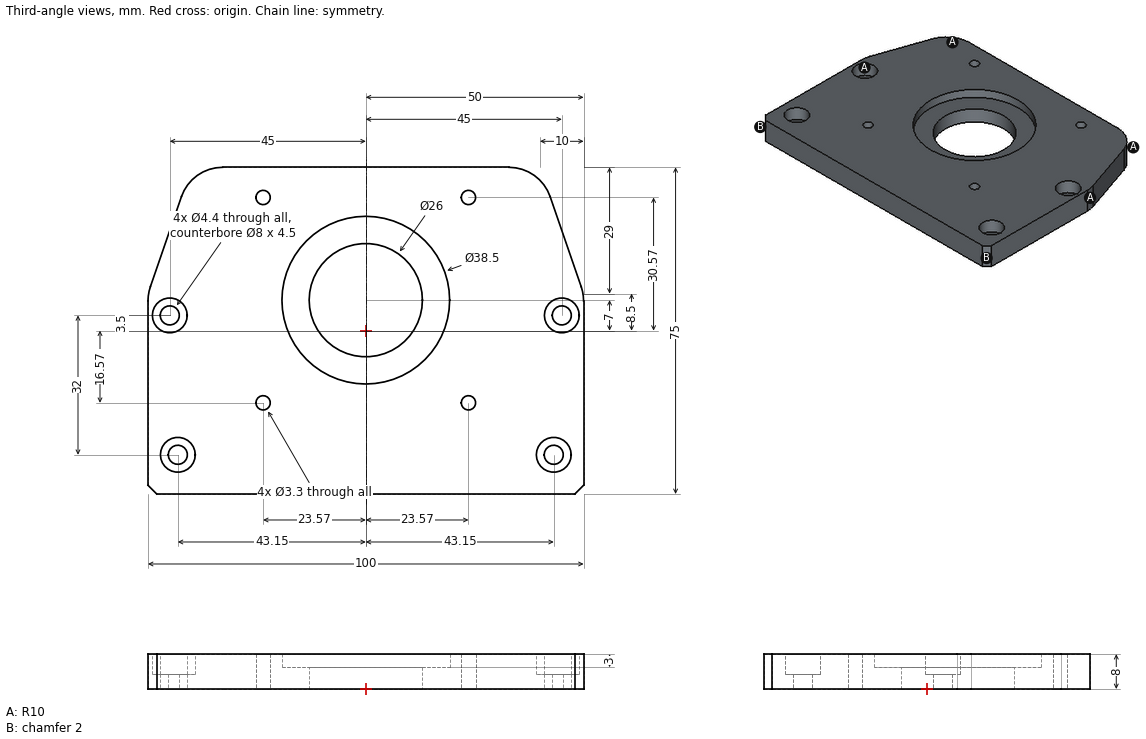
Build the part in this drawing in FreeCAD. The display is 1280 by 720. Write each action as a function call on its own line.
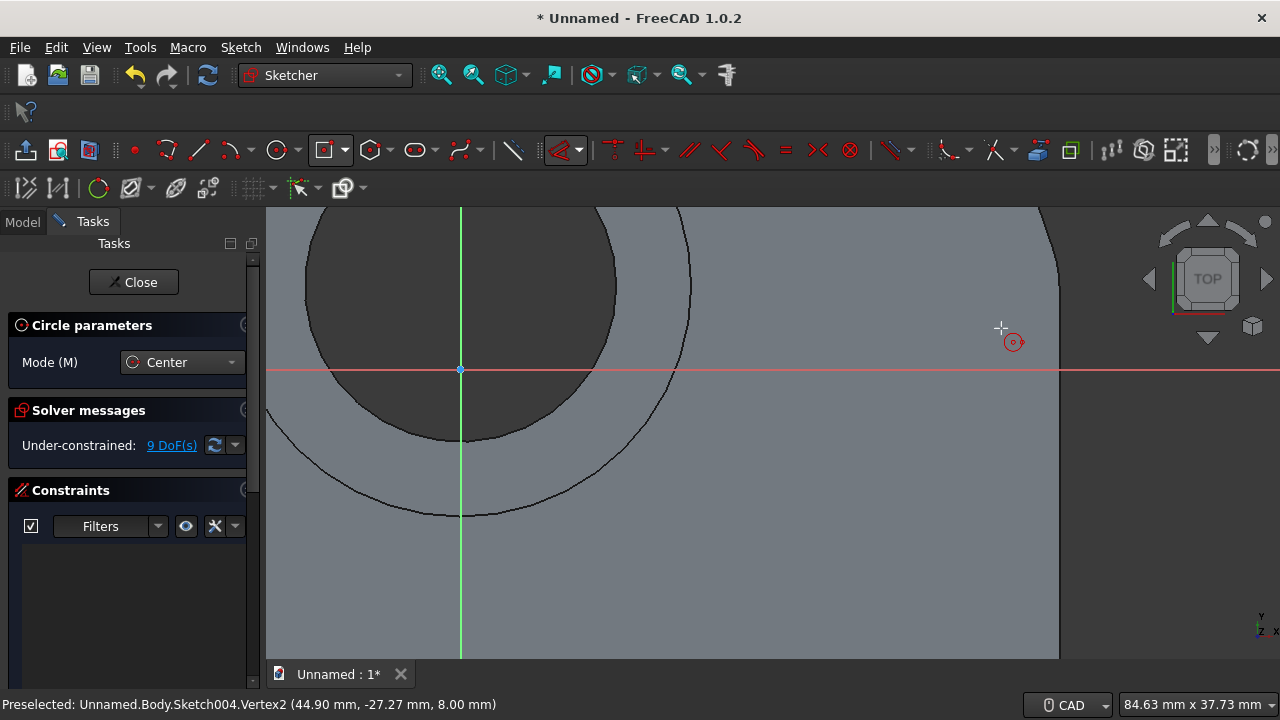
click(1000, 328)
click(1018, 309)
key(Escape)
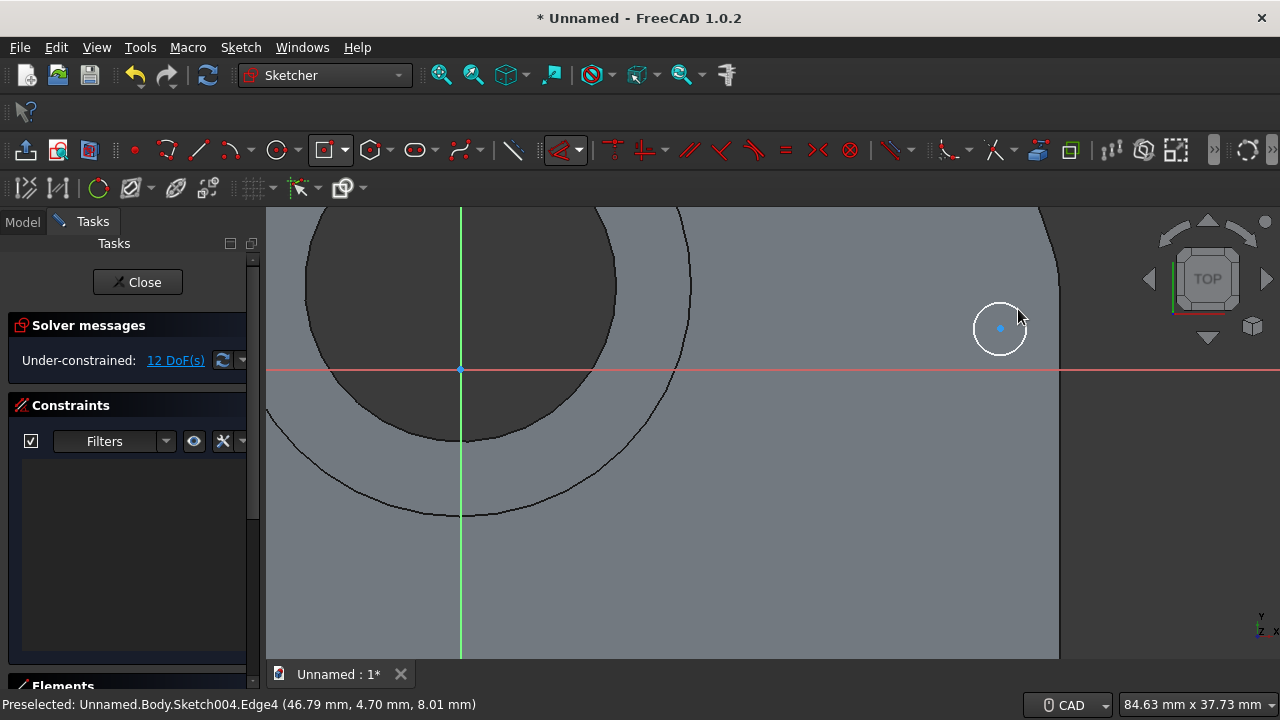
scroll(1001, 328, down, 3)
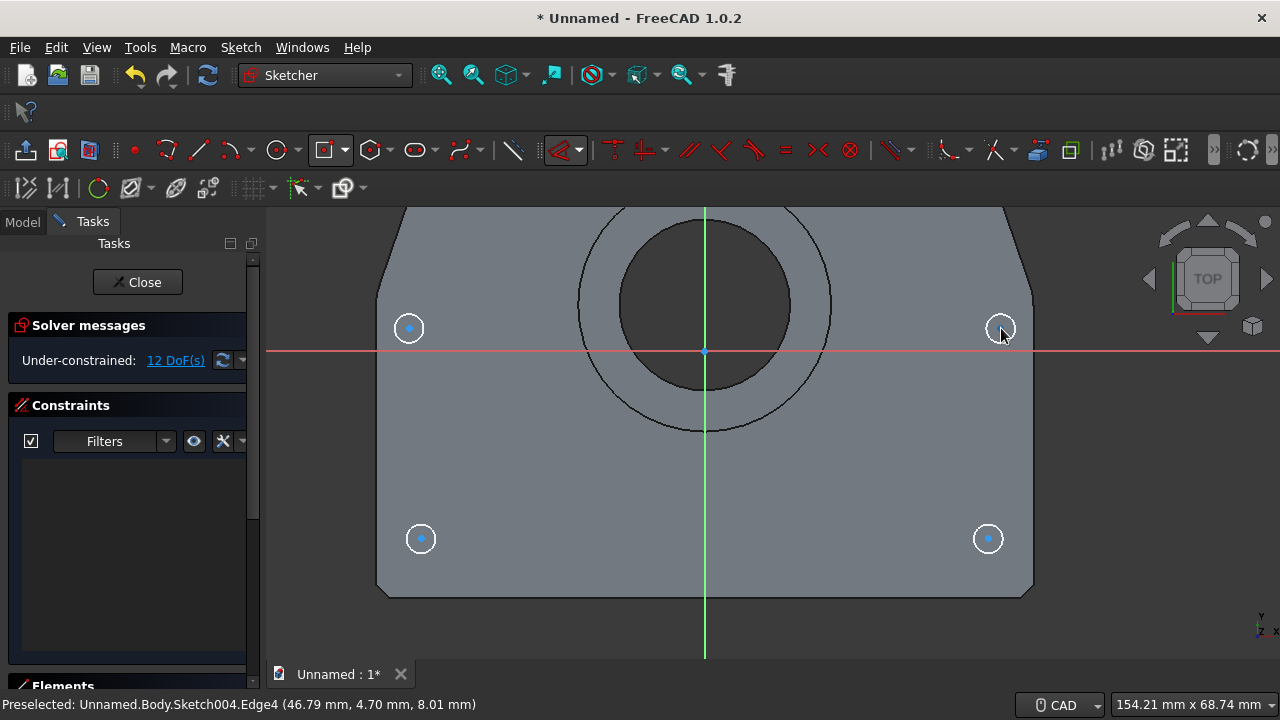
click(419, 318)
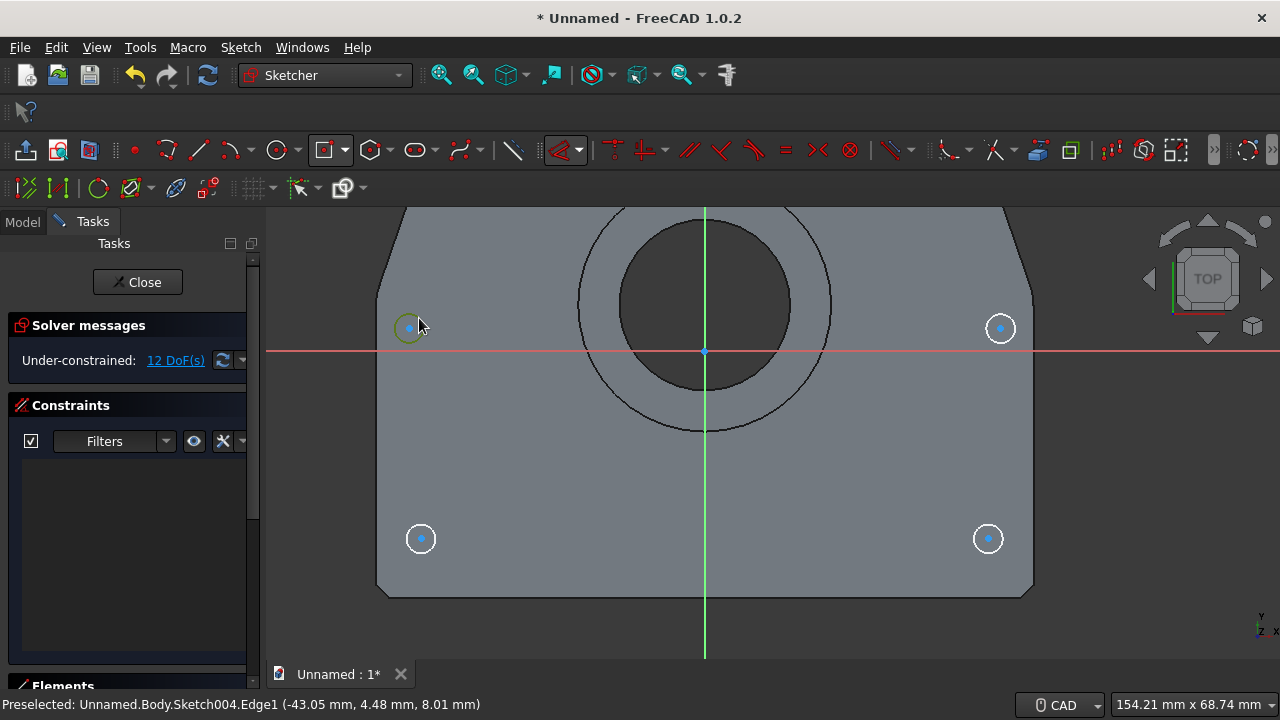
click(431, 529)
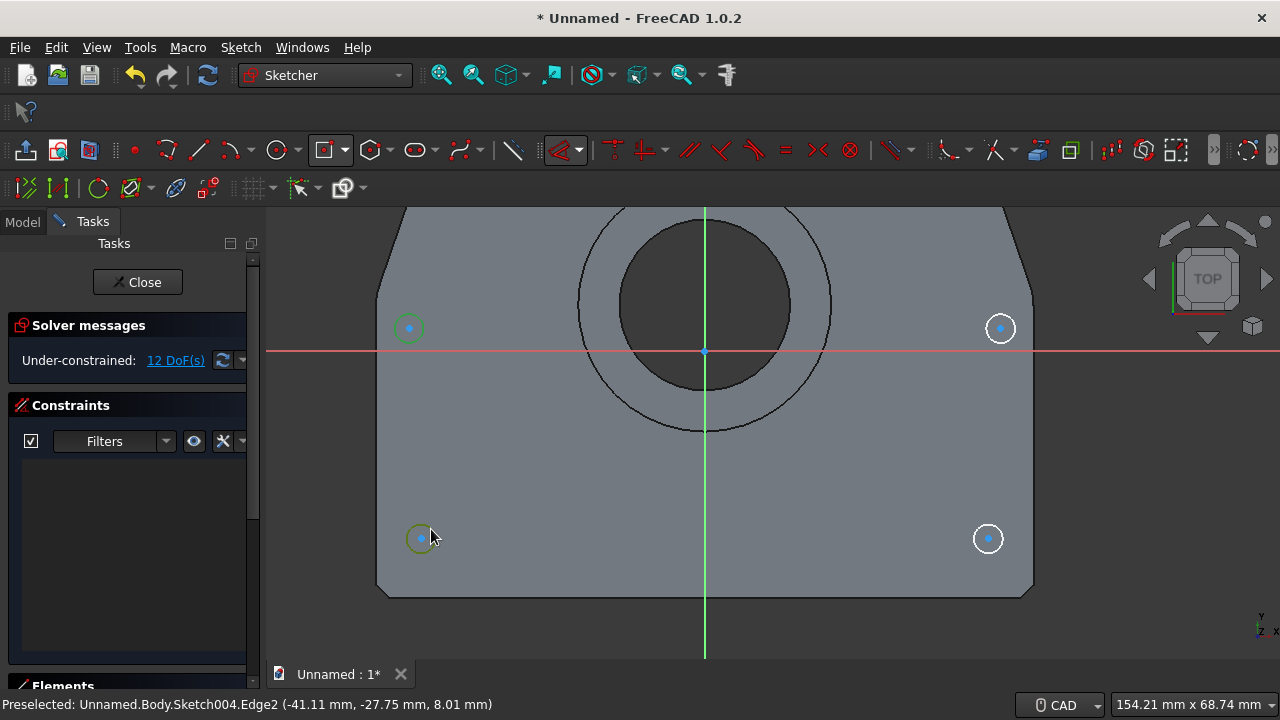
click(998, 529)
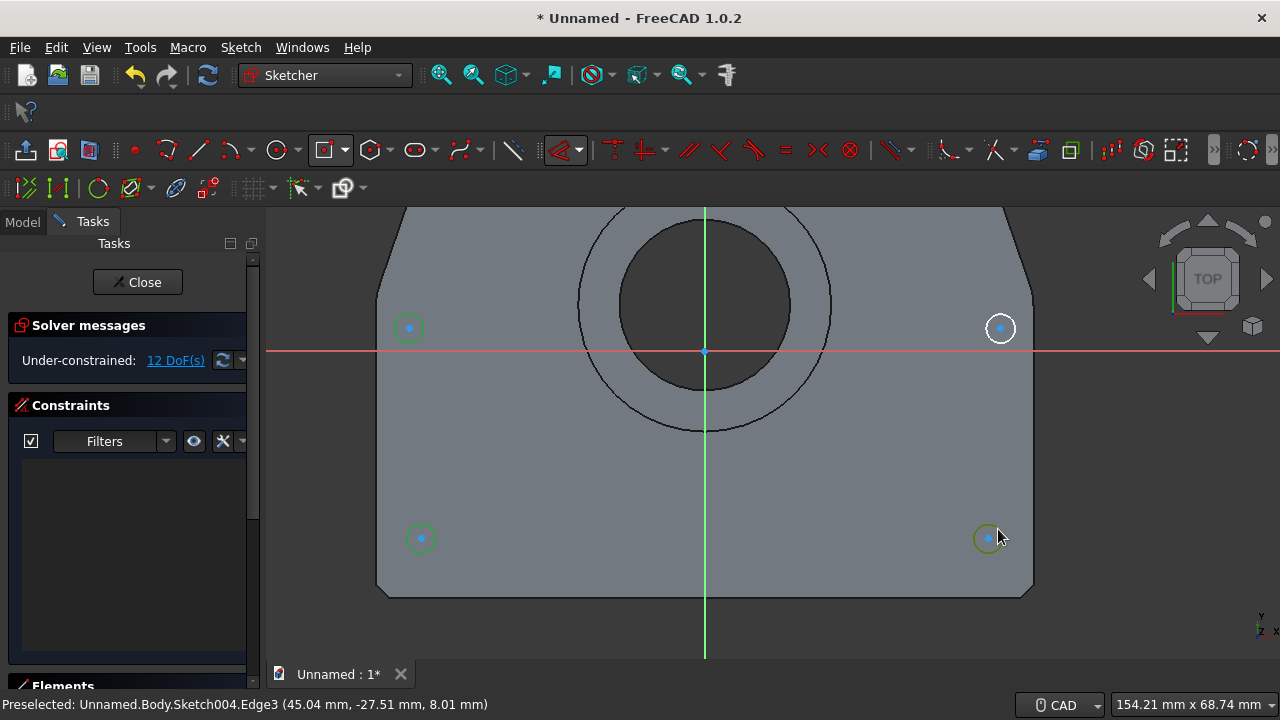
click(1011, 318)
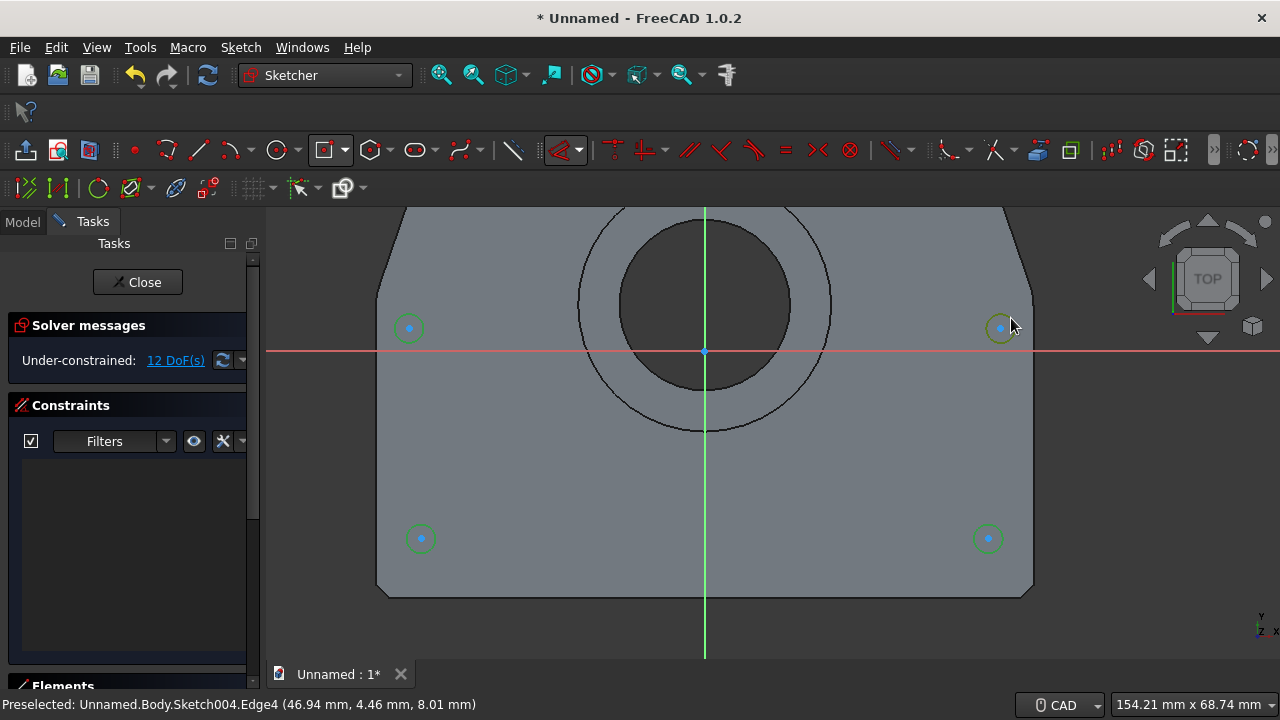
key(e)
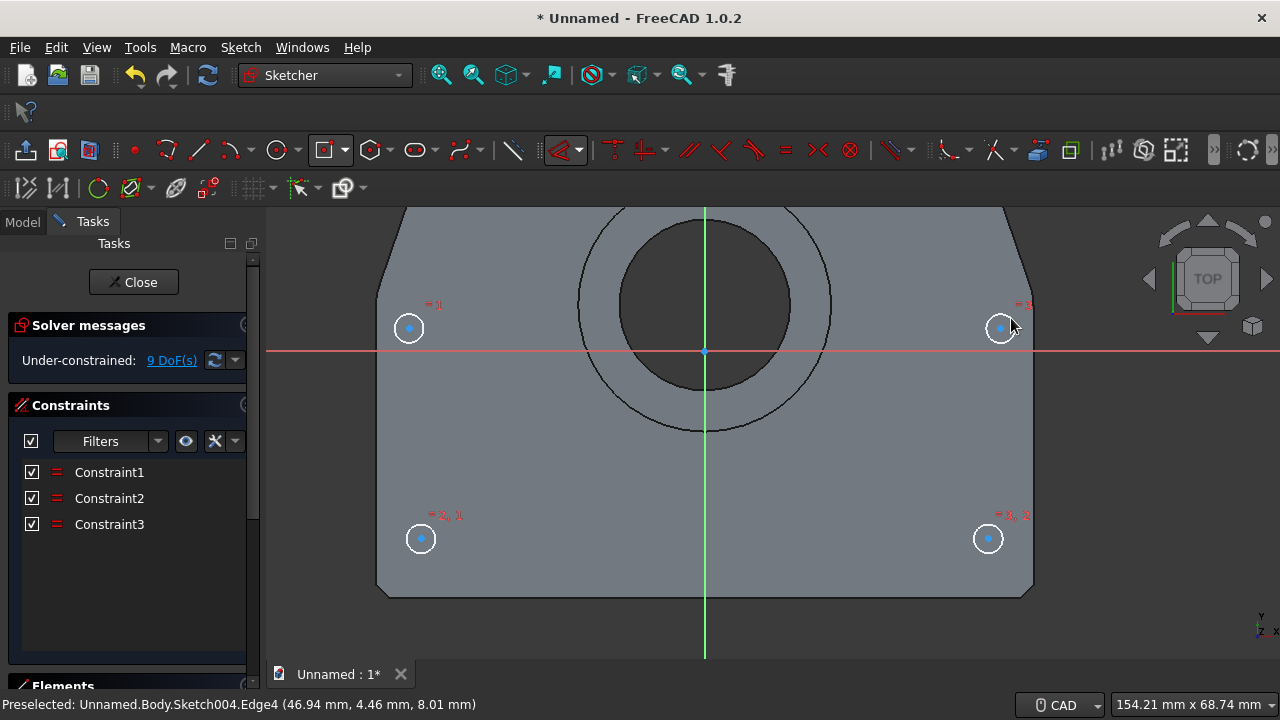
click(421, 539)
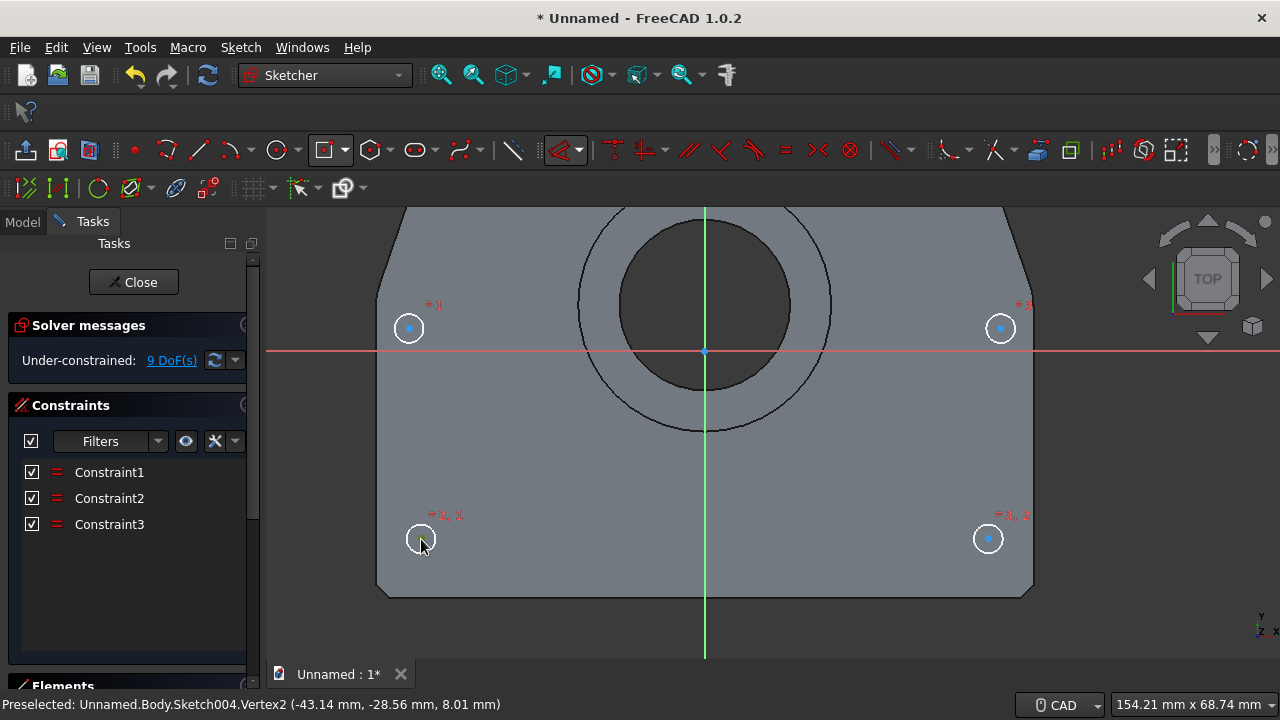
click(988, 539)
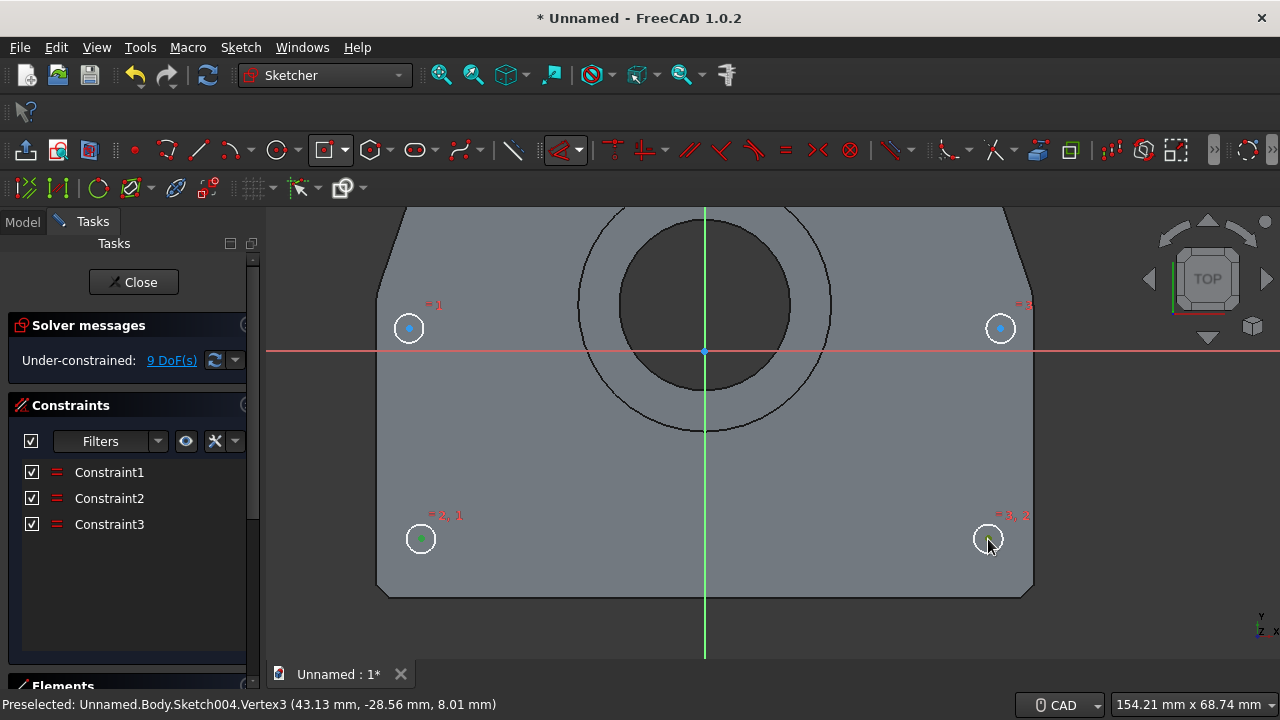
key(h)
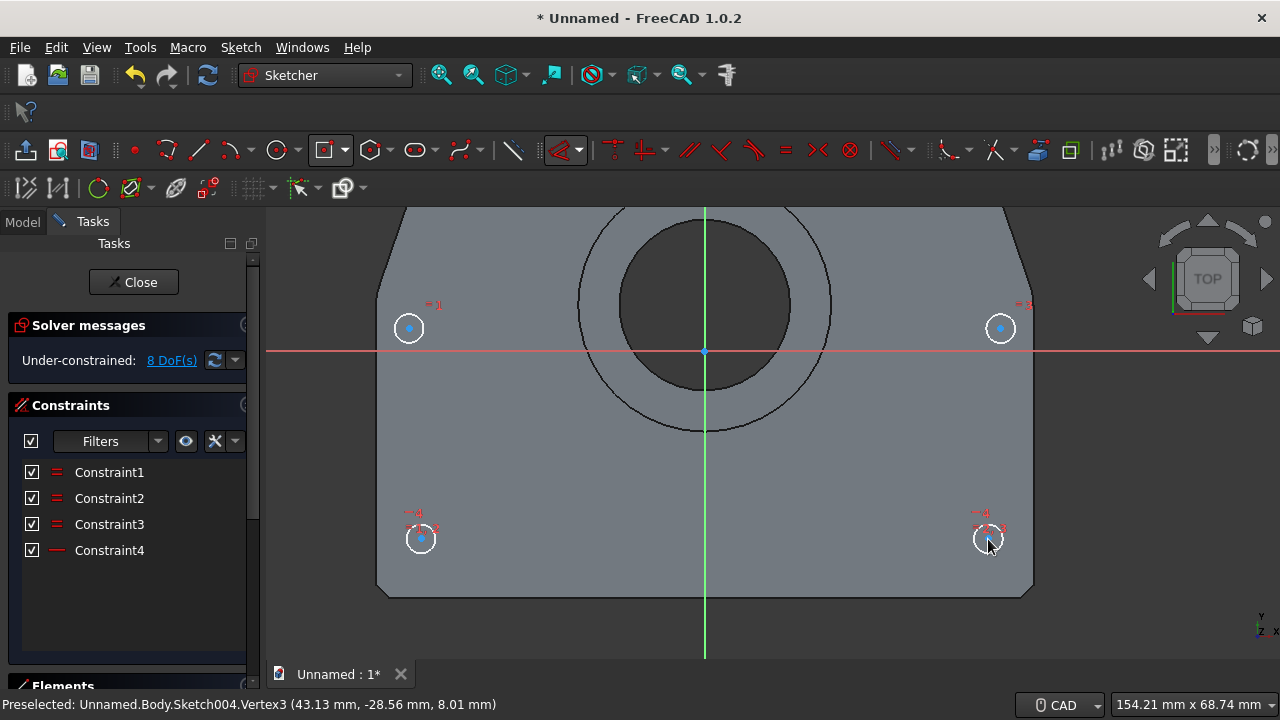
click(409, 329)